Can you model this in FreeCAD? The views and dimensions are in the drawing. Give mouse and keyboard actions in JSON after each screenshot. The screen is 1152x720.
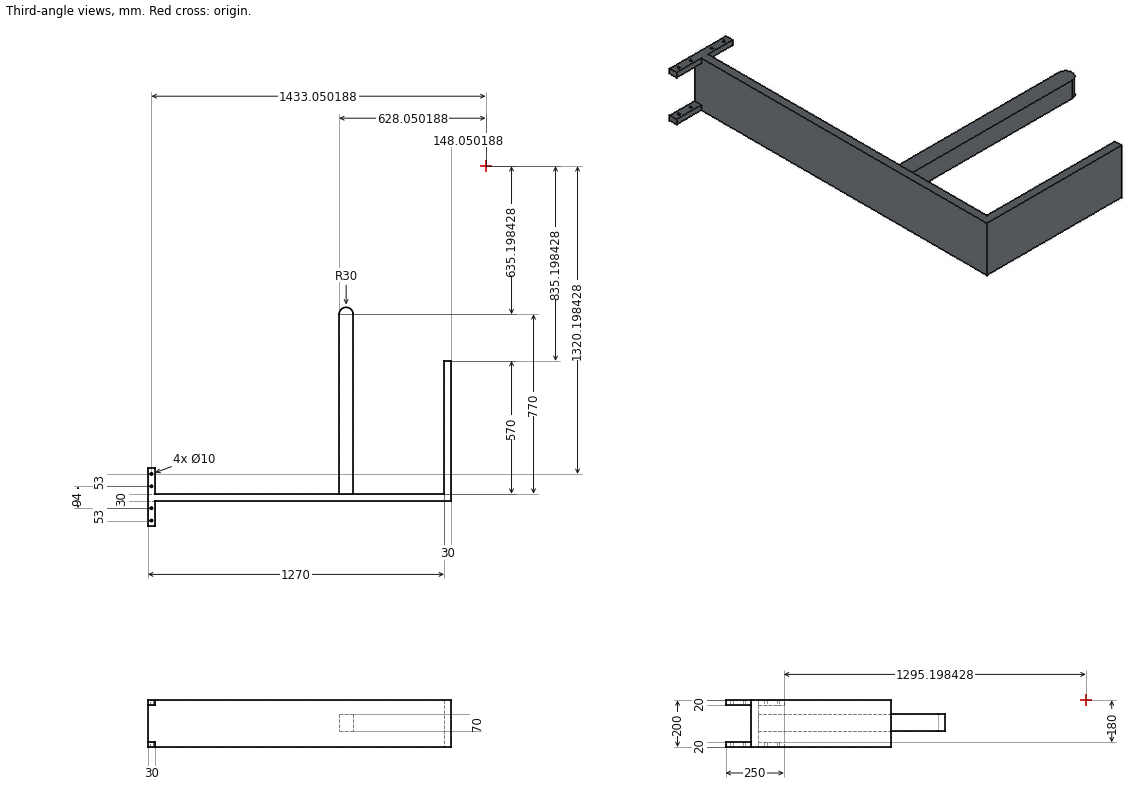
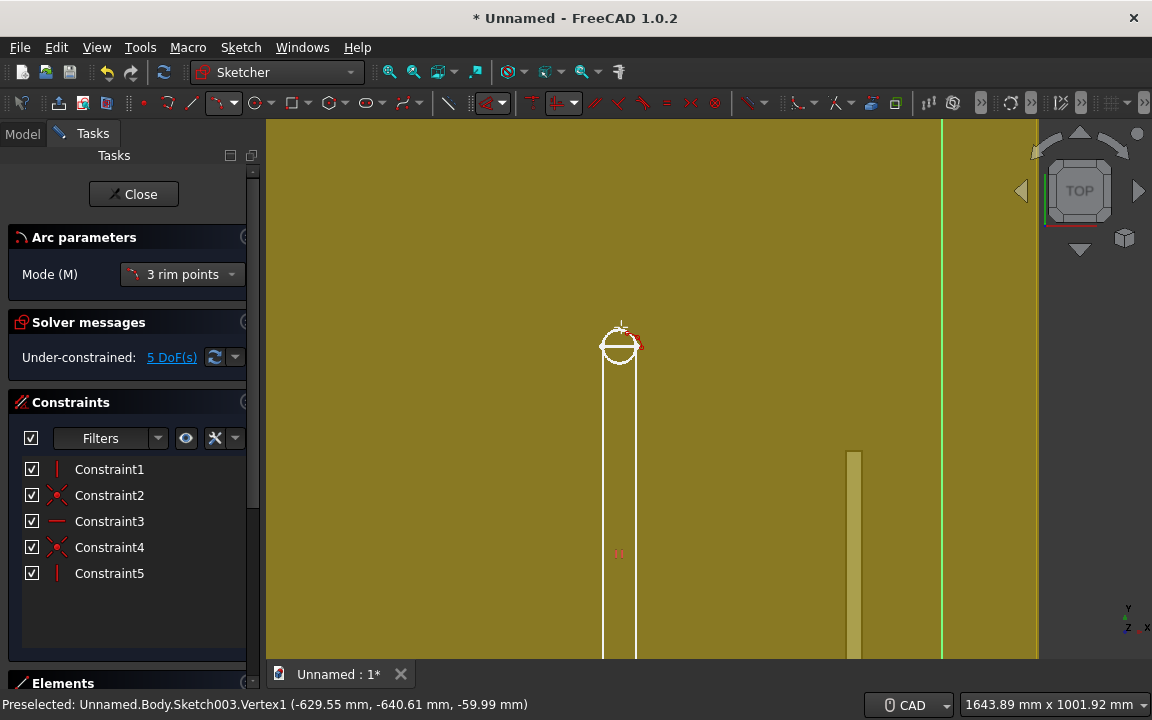
{"action": "left_click", "coordinate": [620, 327]}
{"action": "key", "text": "Escape"}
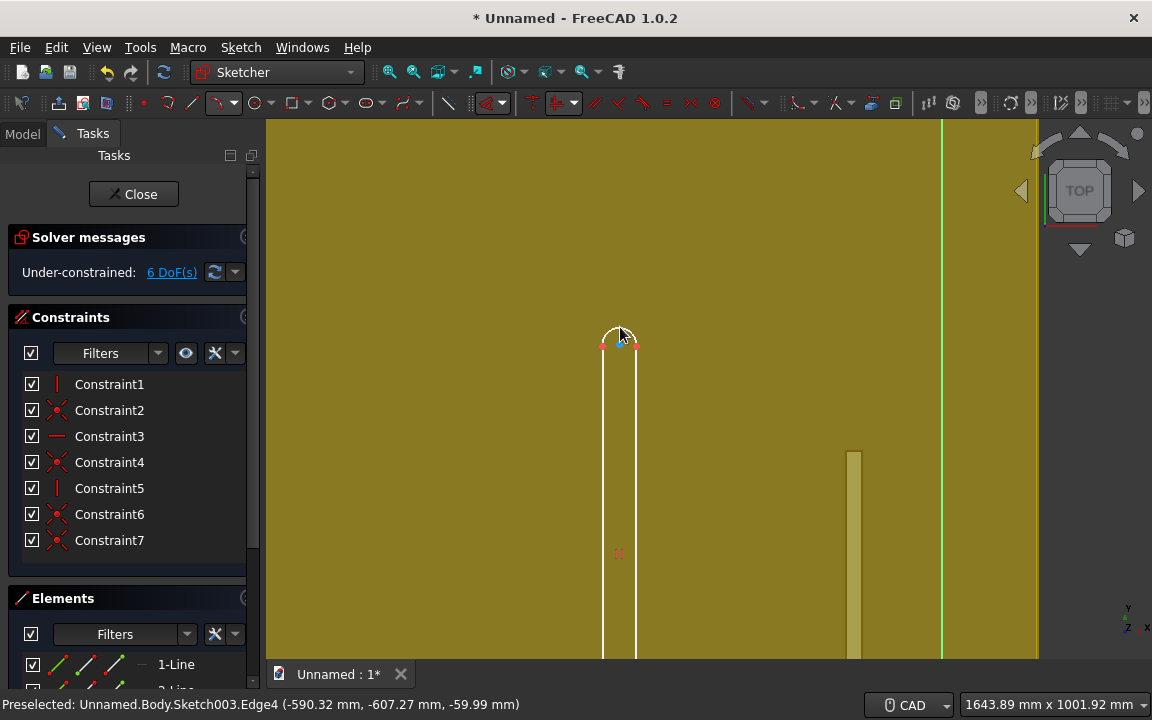
{"action": "left_click", "coordinate": [603, 471]}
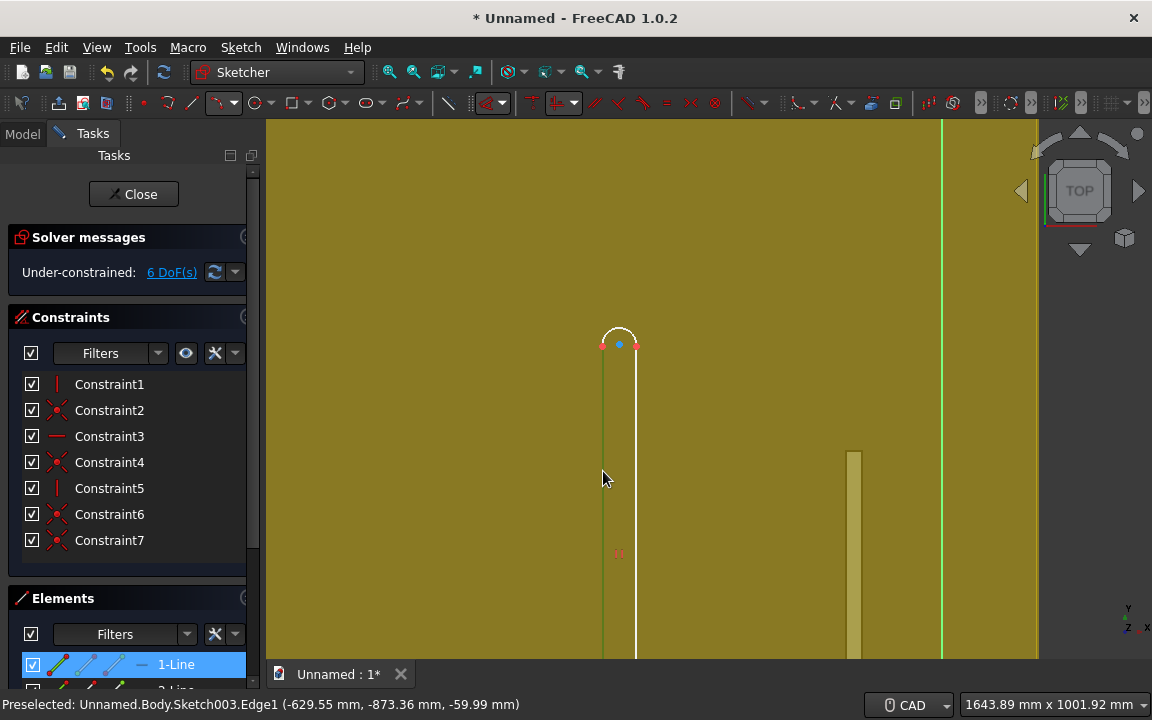
{"action": "left_click", "coordinate": [630, 332]}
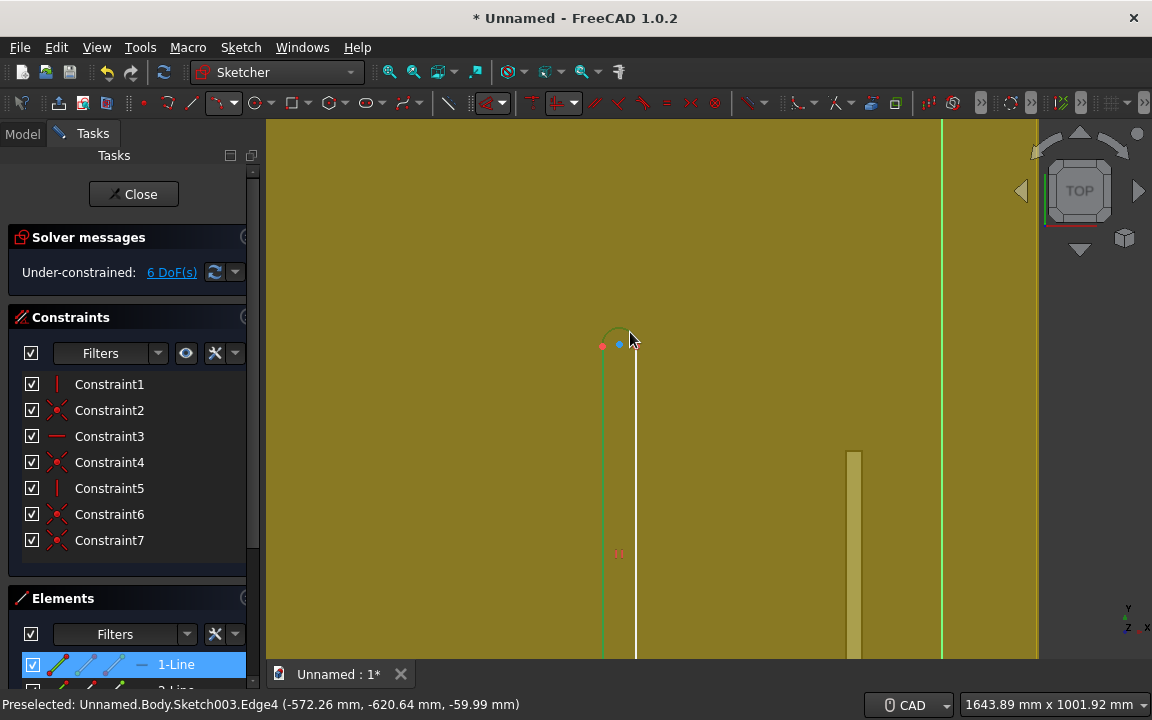
{"action": "left_click", "coordinate": [644, 104]}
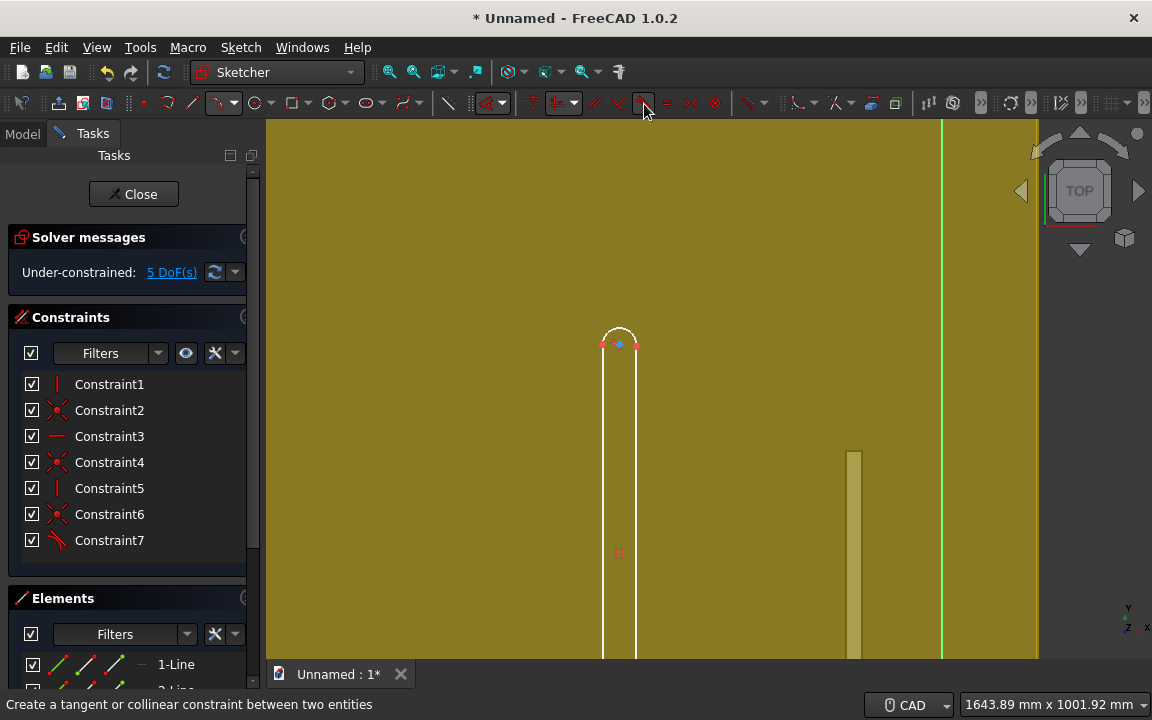
{"action": "left_click", "coordinate": [636, 471]}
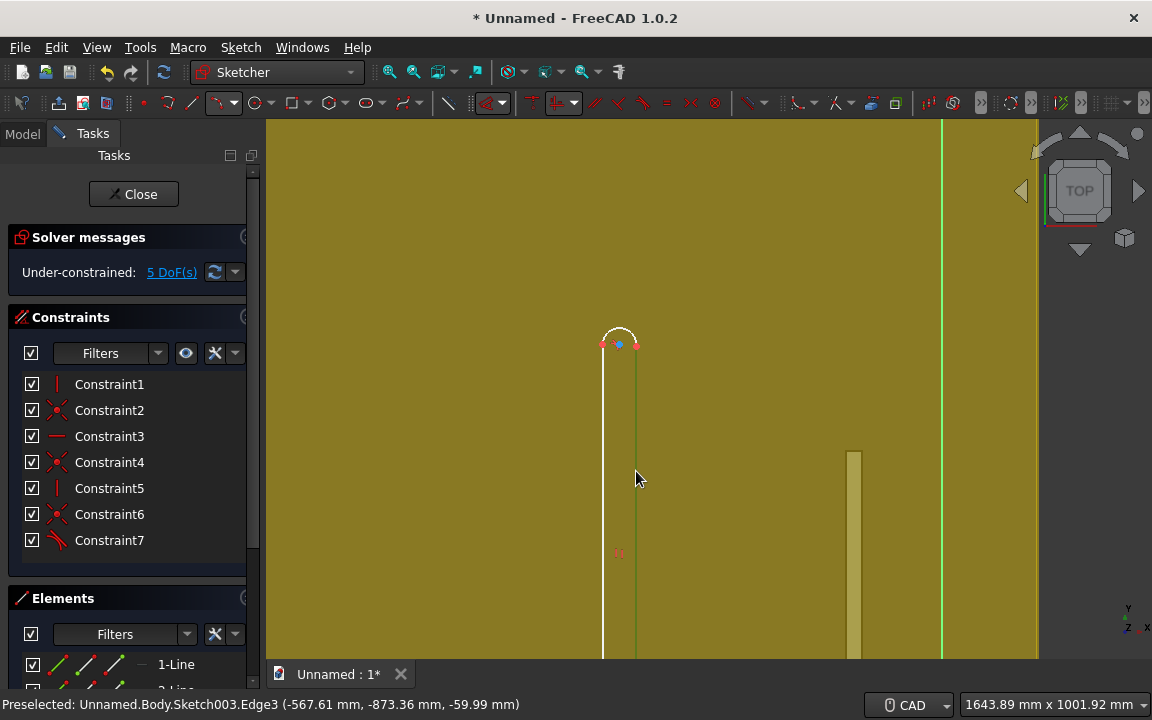
{"action": "left_click", "coordinate": [630, 332]}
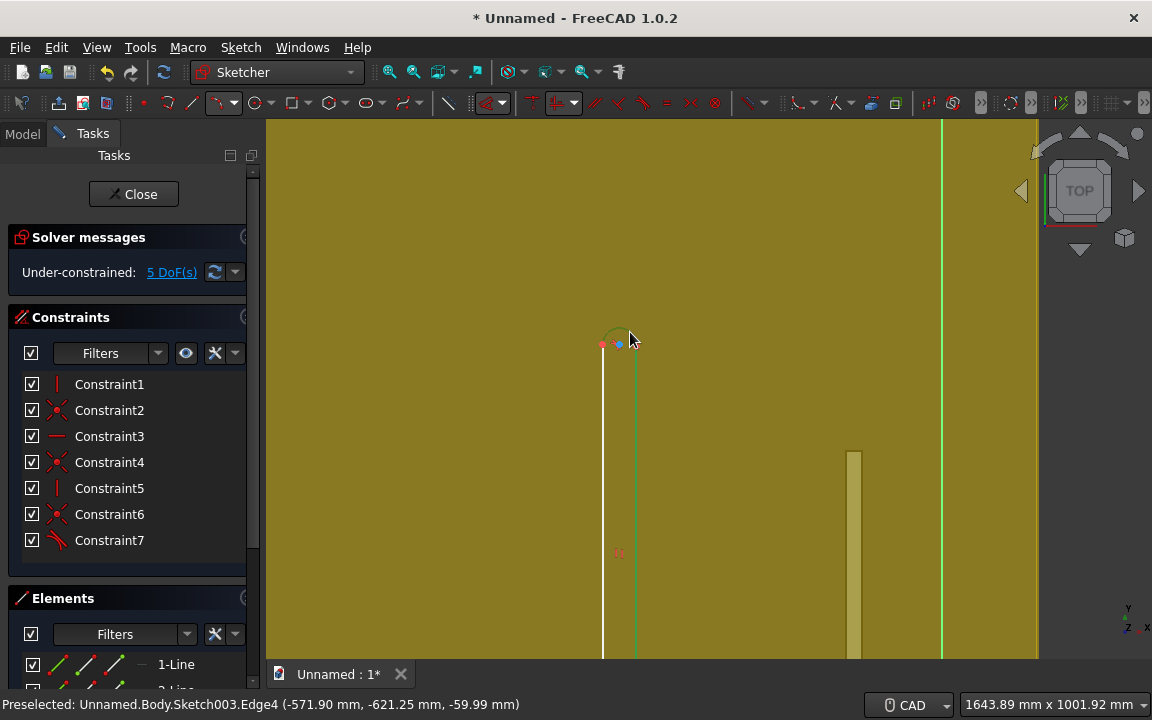
{"action": "left_click", "coordinate": [644, 104]}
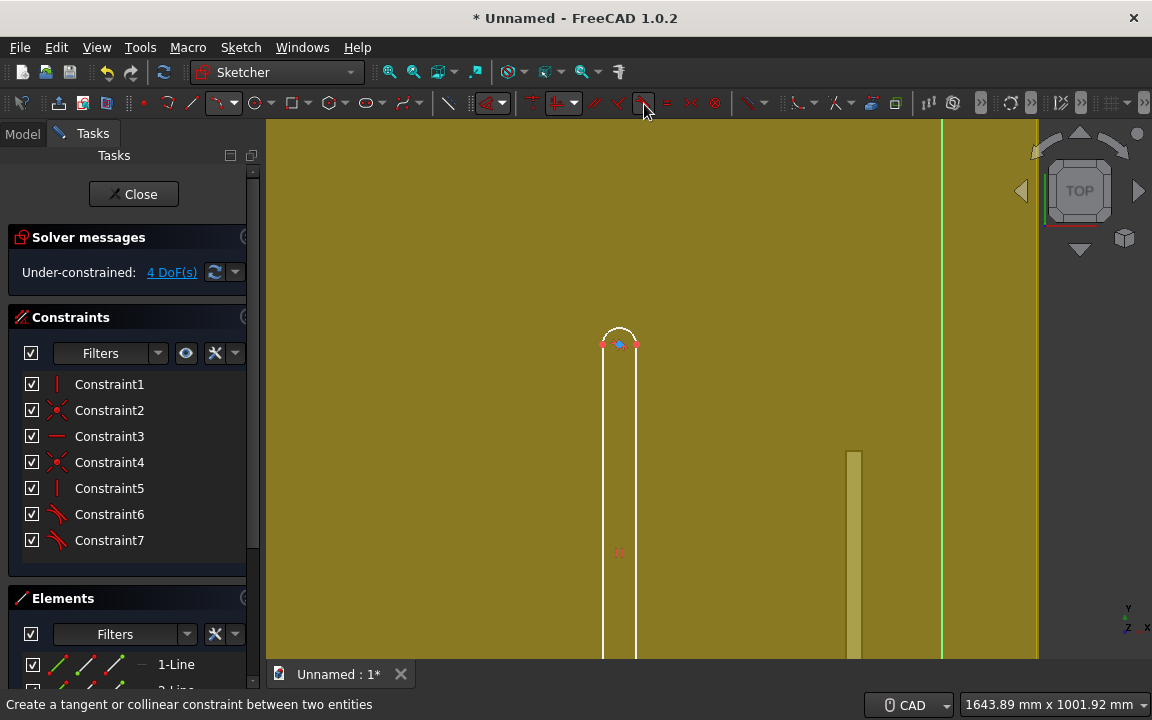
{"action": "scroll", "coordinate": [629, 331], "scroll_direction": "up", "scroll_amount": 5}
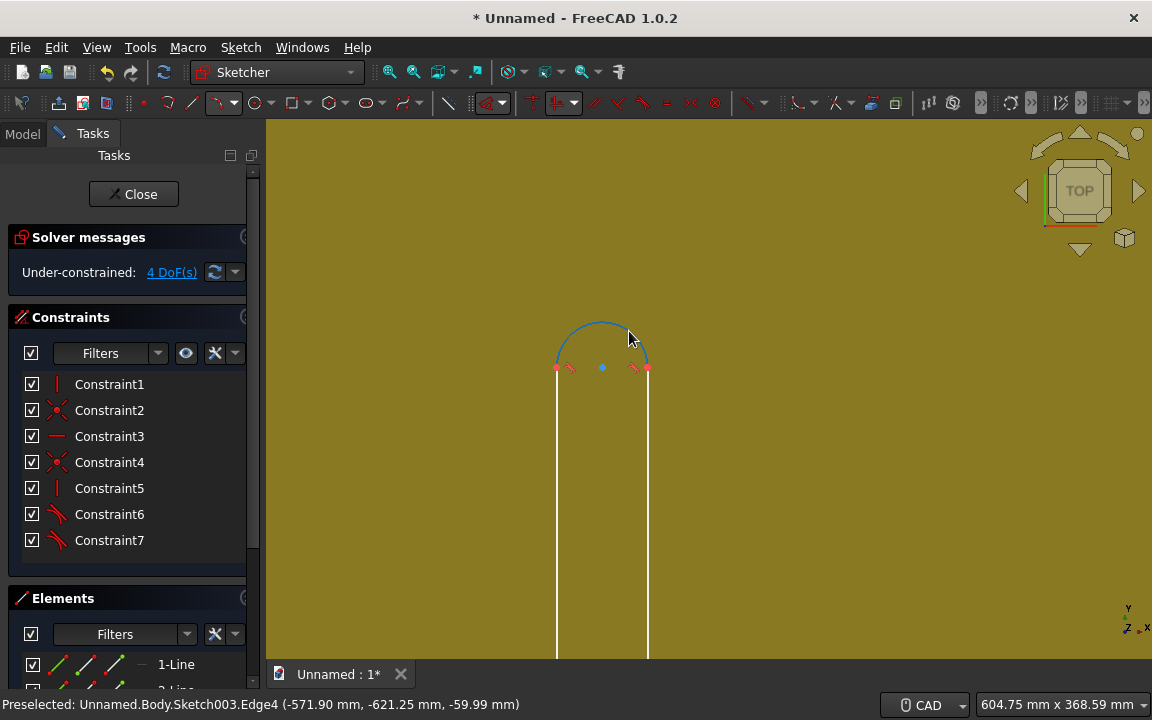
{"action": "left_click", "coordinate": [629, 331]}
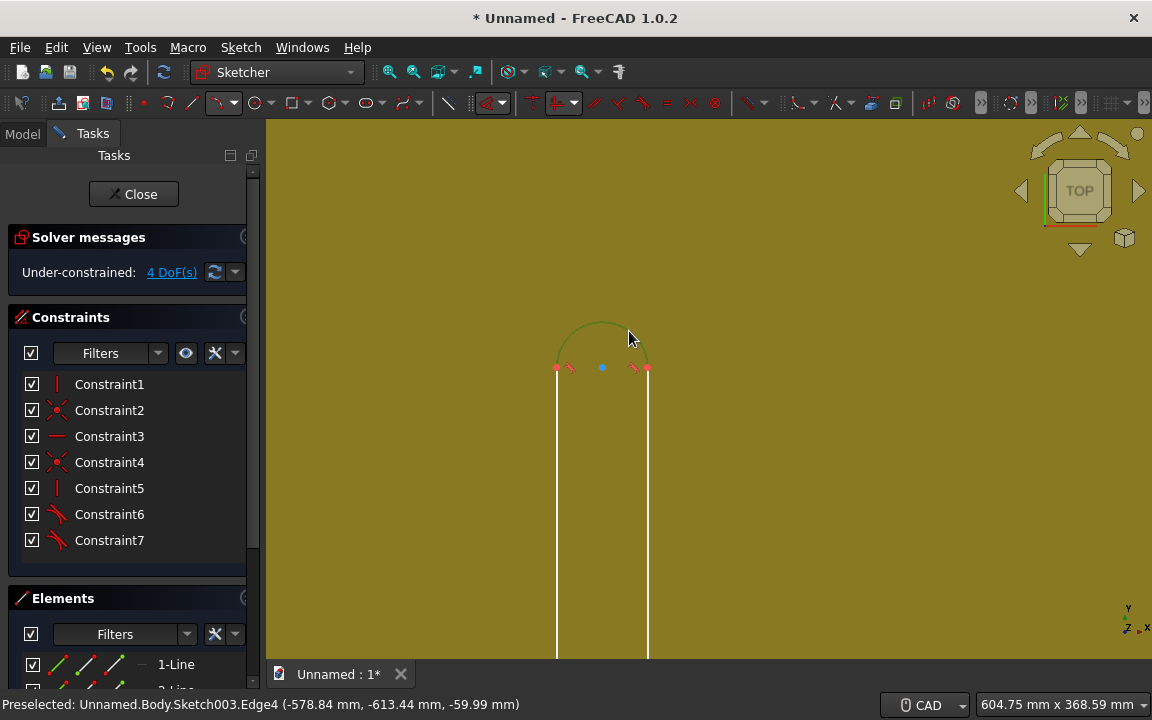
{"action": "left_click", "coordinate": [504, 104]}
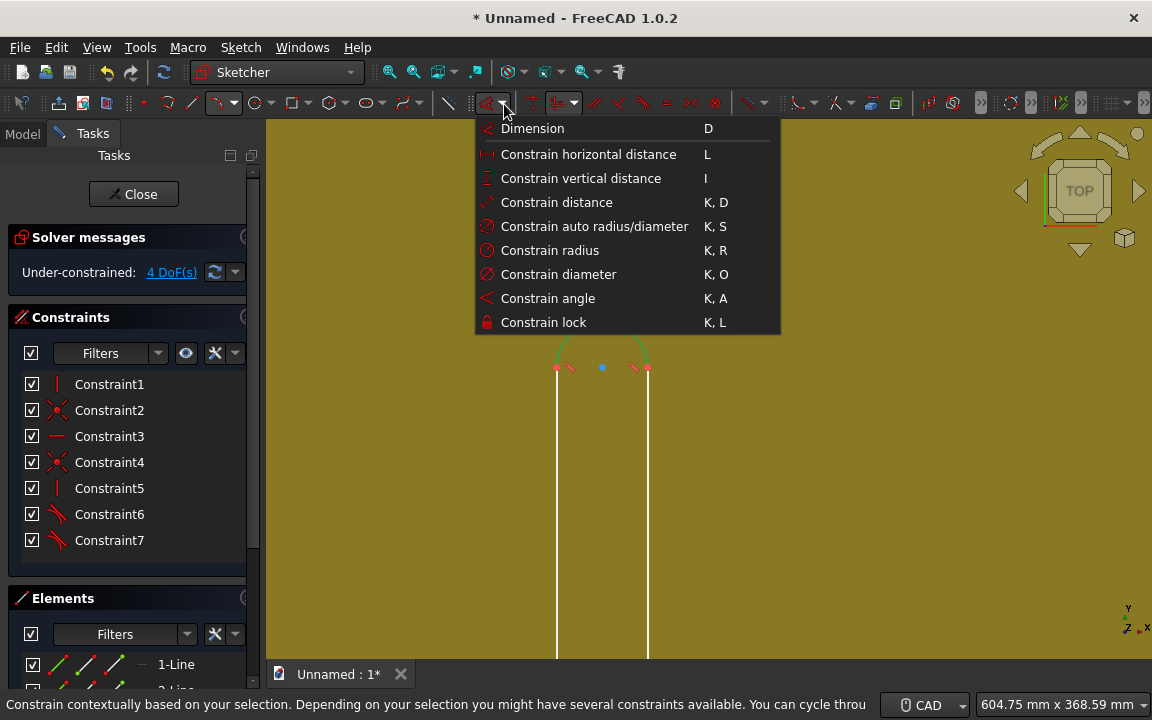
{"action": "left_click", "coordinate": [628, 250]}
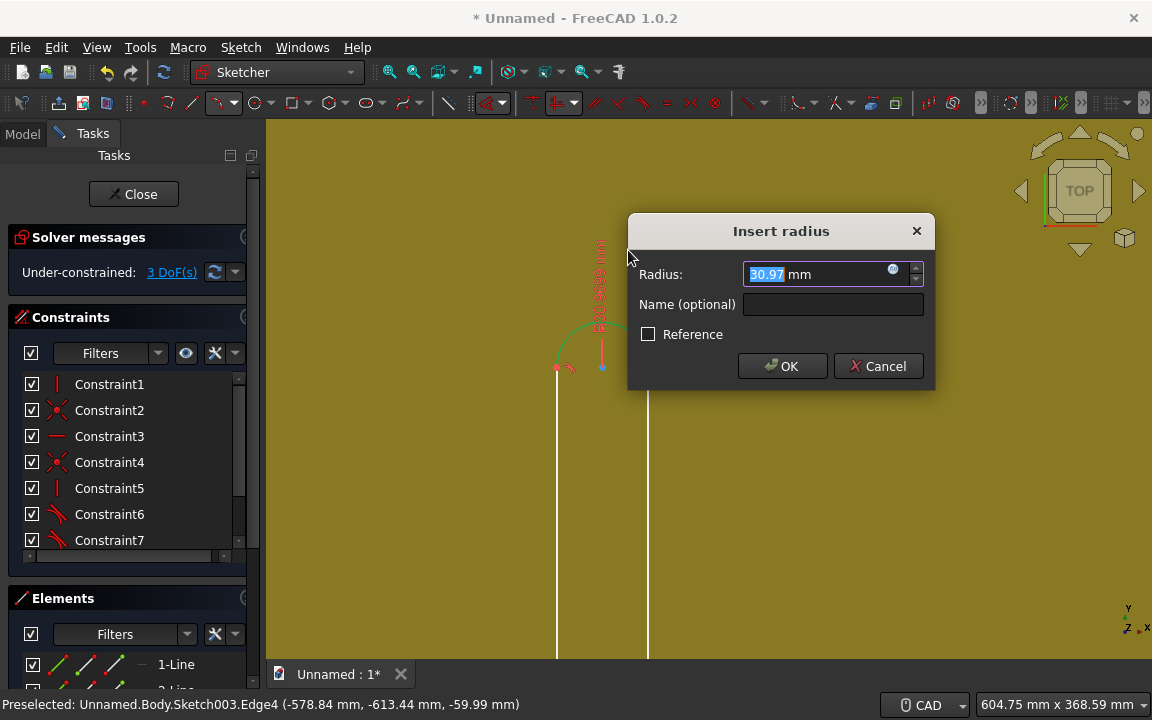
{"action": "type", "text": "30"}
{"action": "key", "text": "Return"}